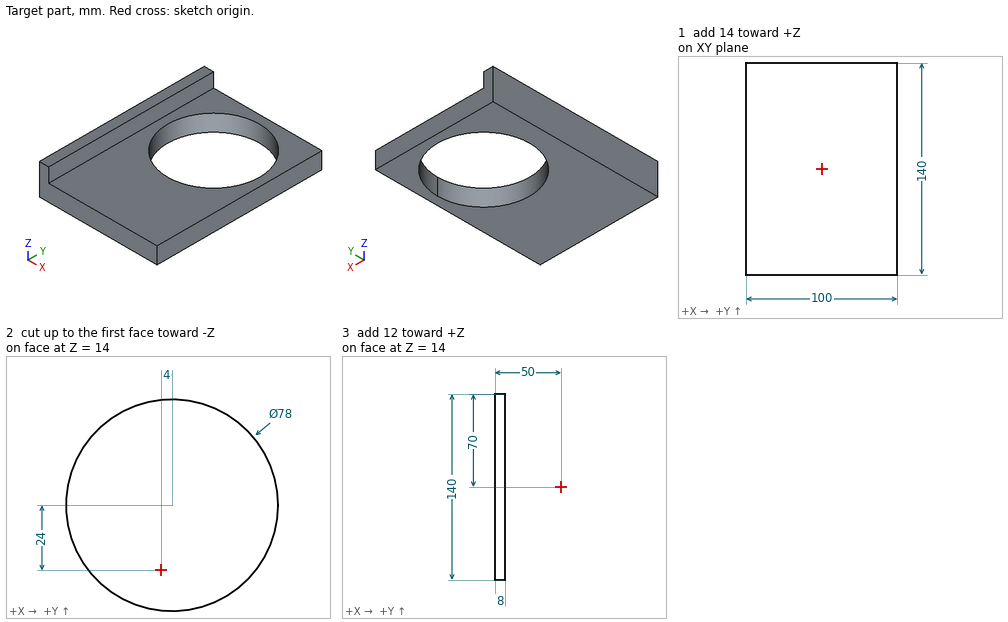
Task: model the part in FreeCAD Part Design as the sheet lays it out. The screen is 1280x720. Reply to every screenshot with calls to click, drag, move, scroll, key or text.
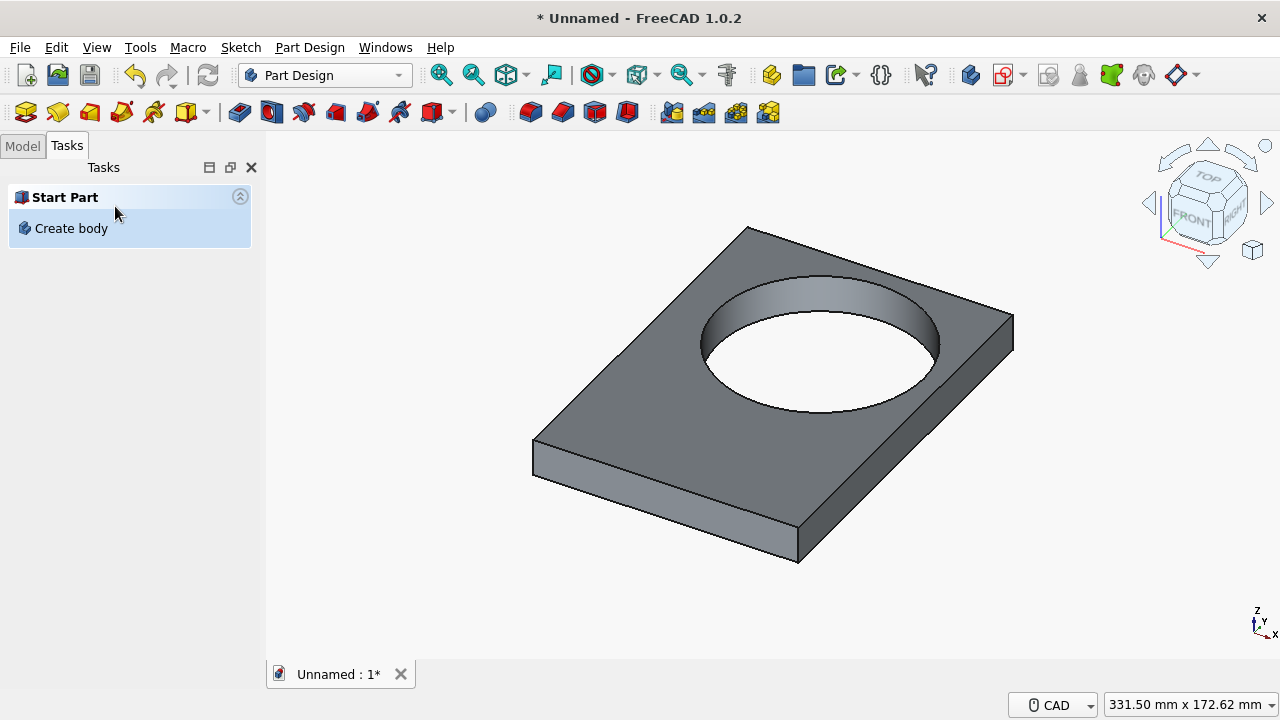
click(674, 425)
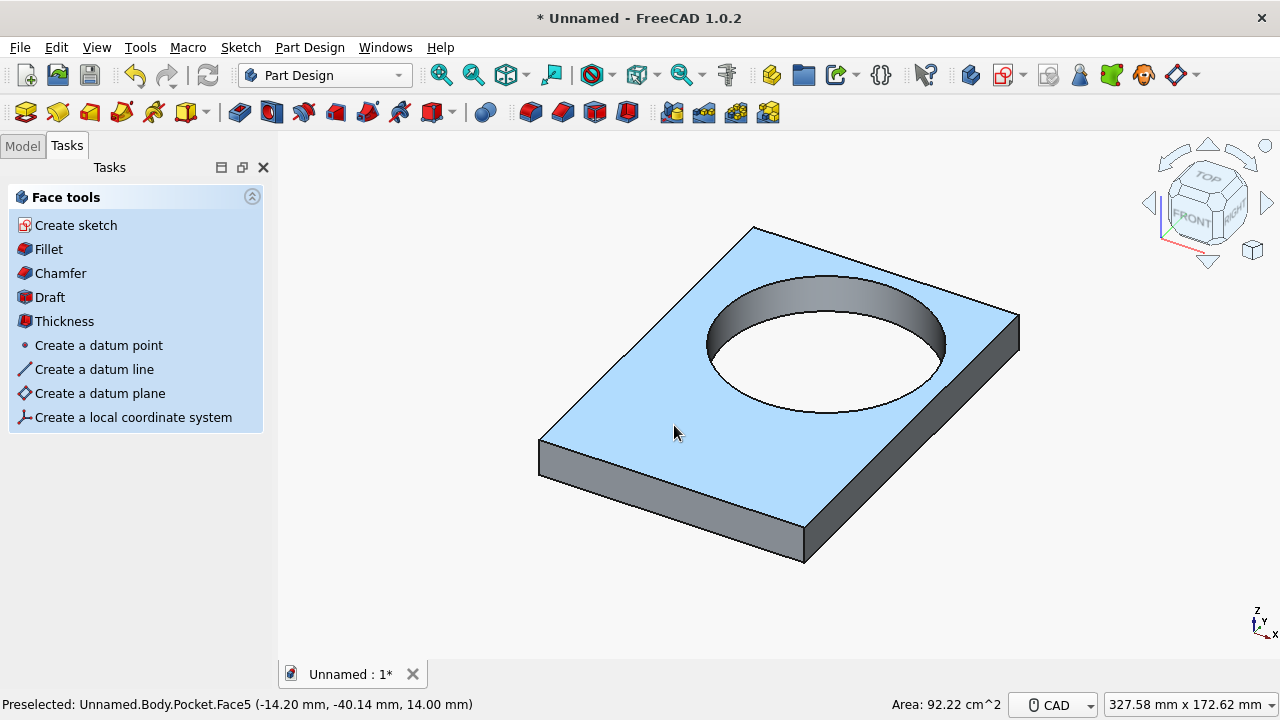
click(1004, 76)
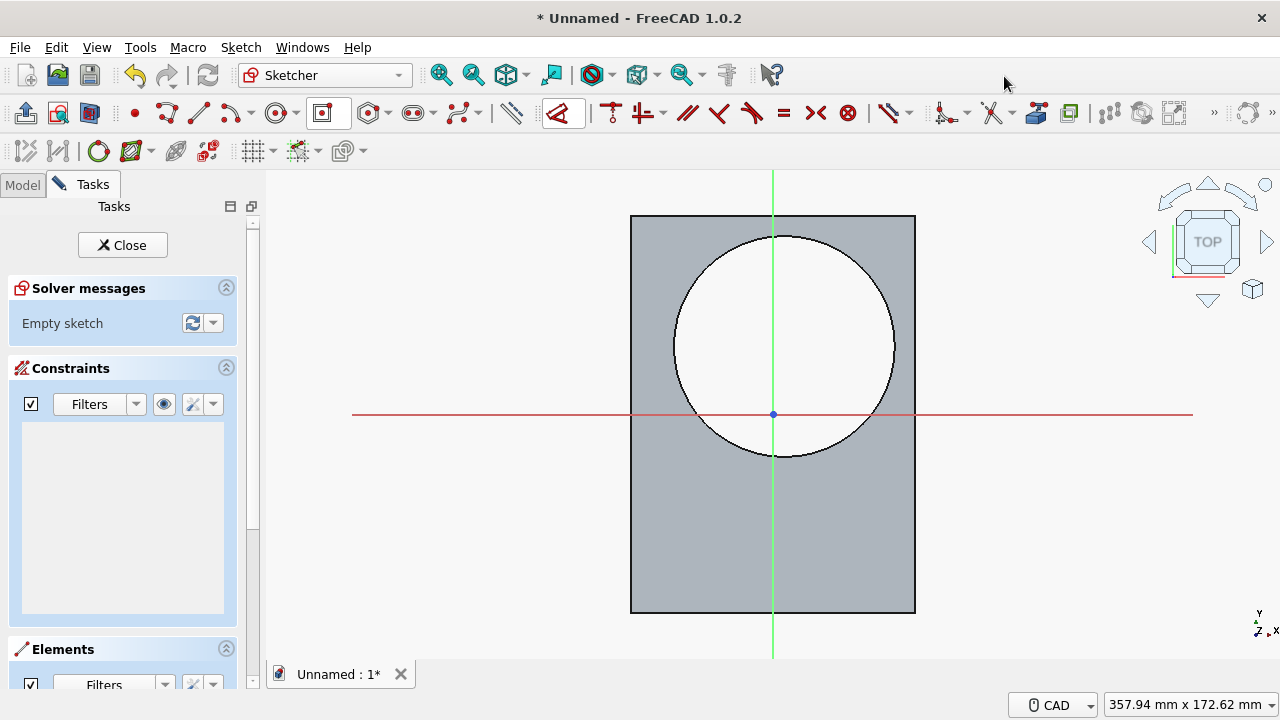
scroll(715, 415, down, 1)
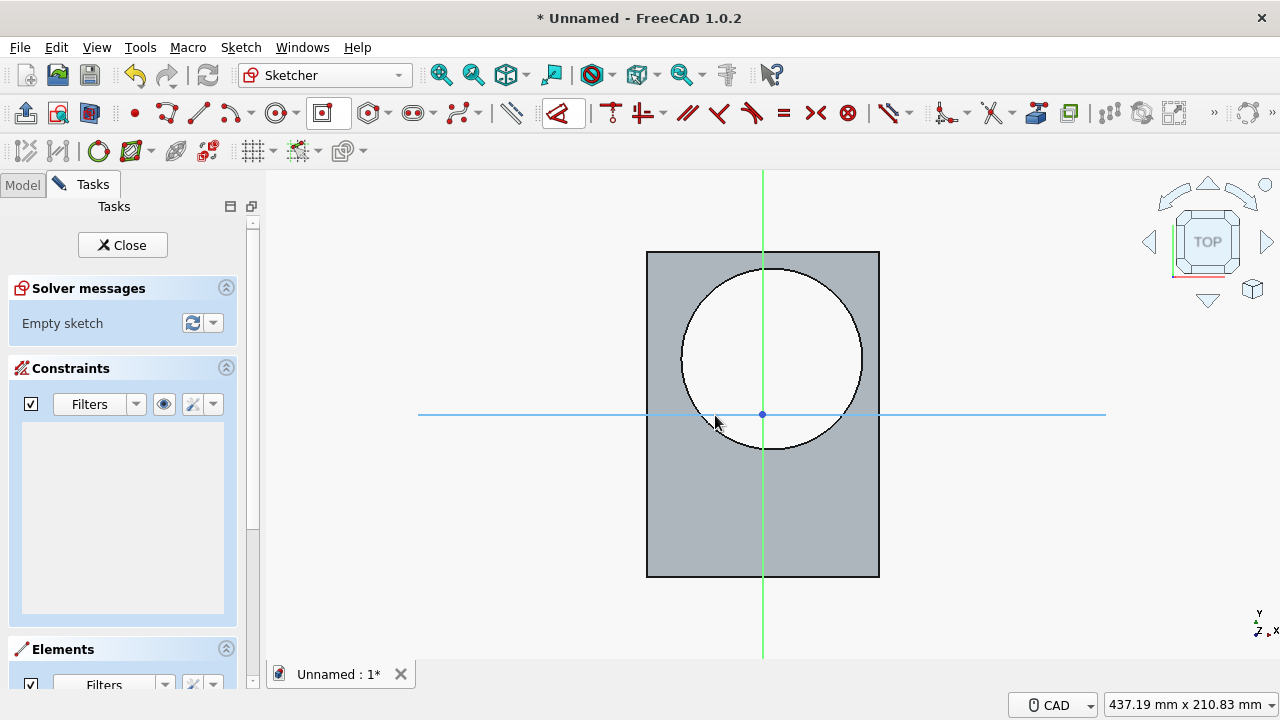
click(346, 114)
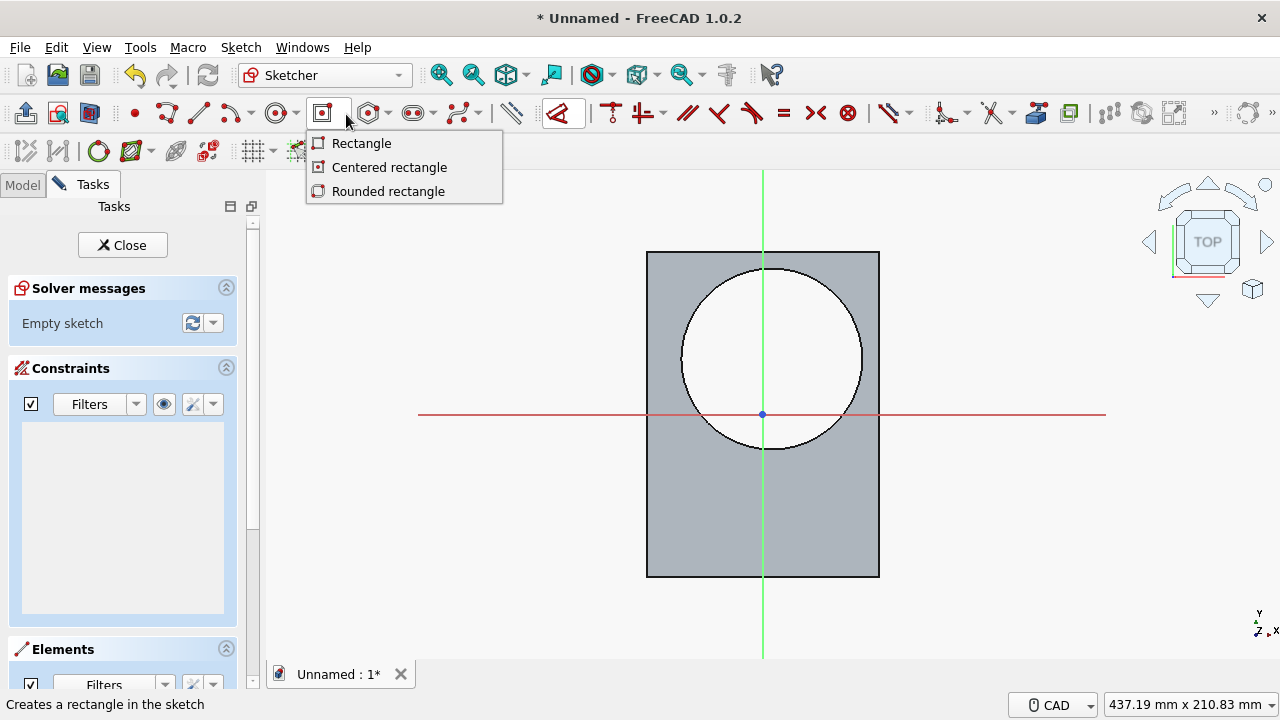
click(404, 143)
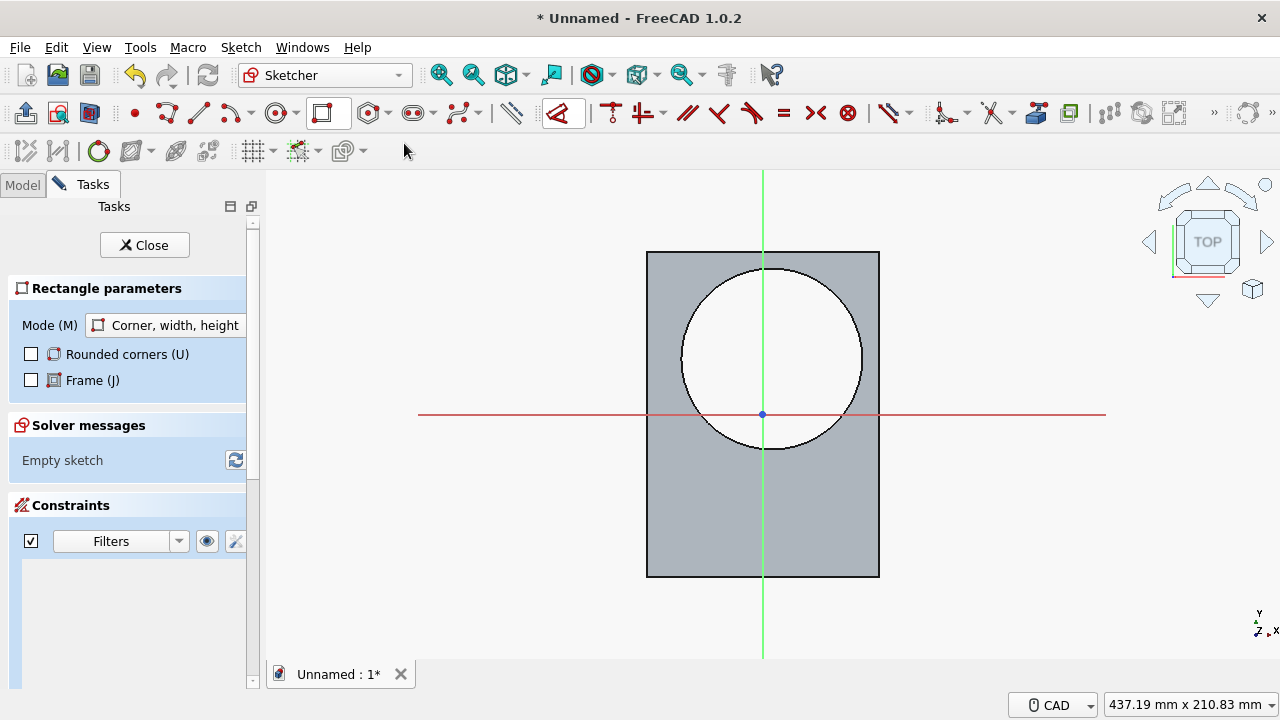
click(647, 252)
move(665, 577)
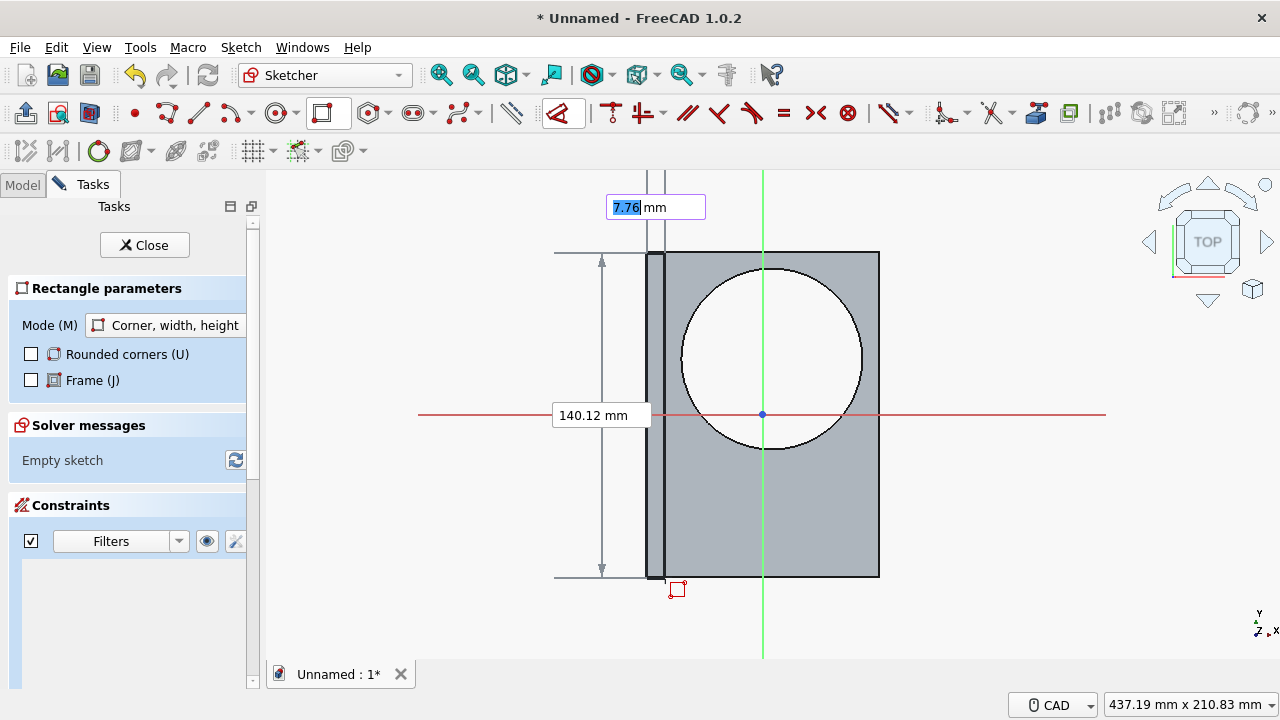
text(8)
key(Tab)
text(140)
key(Return)
key(Escape)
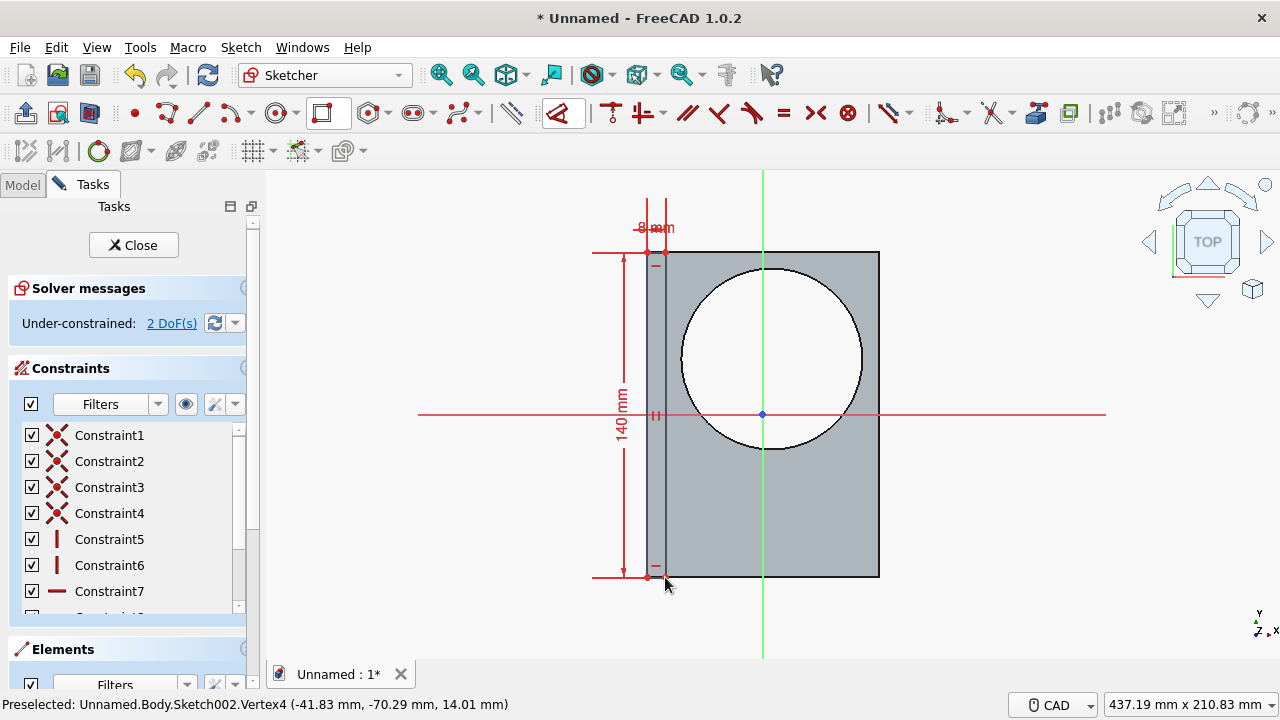
click(647, 253)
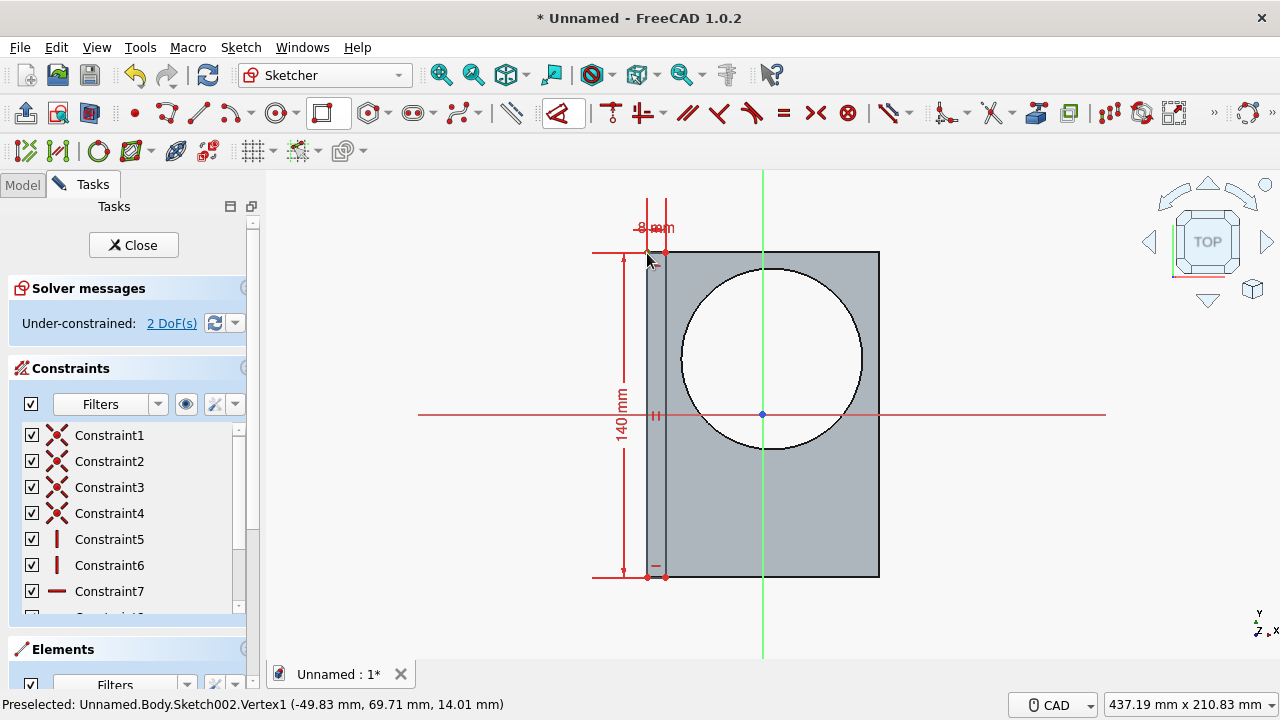
key(l)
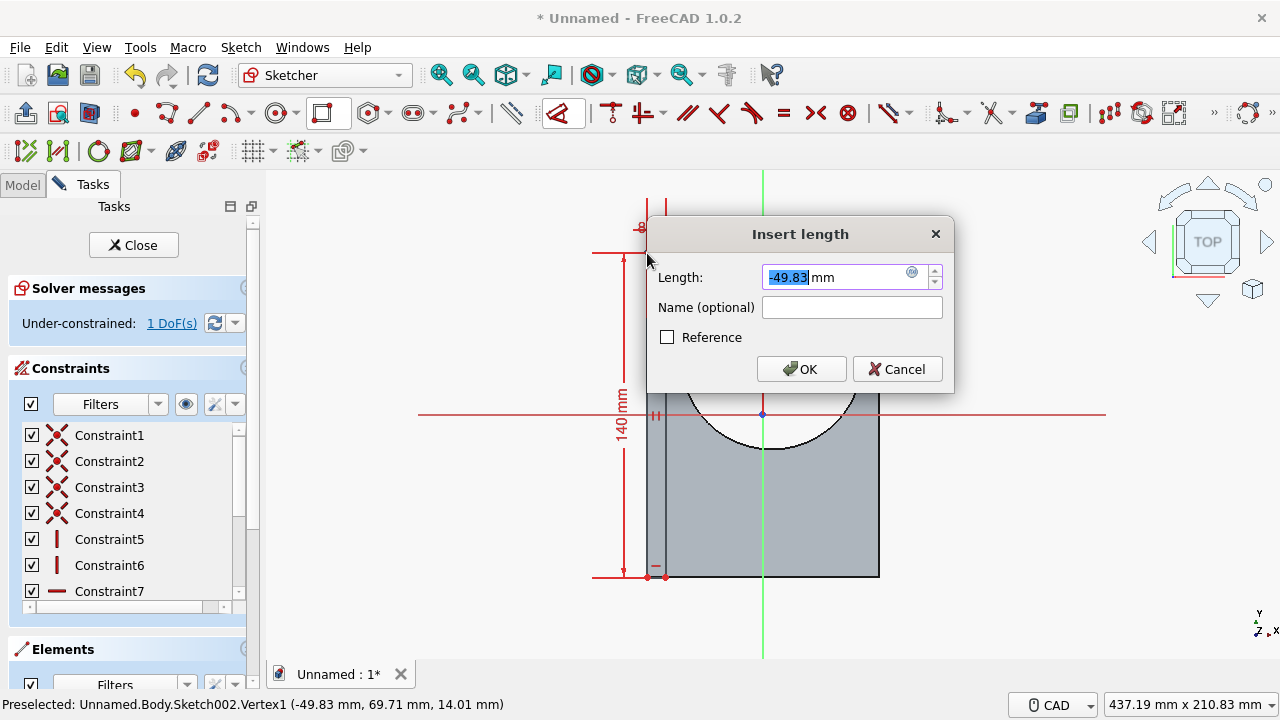
text(-50)
key(Return)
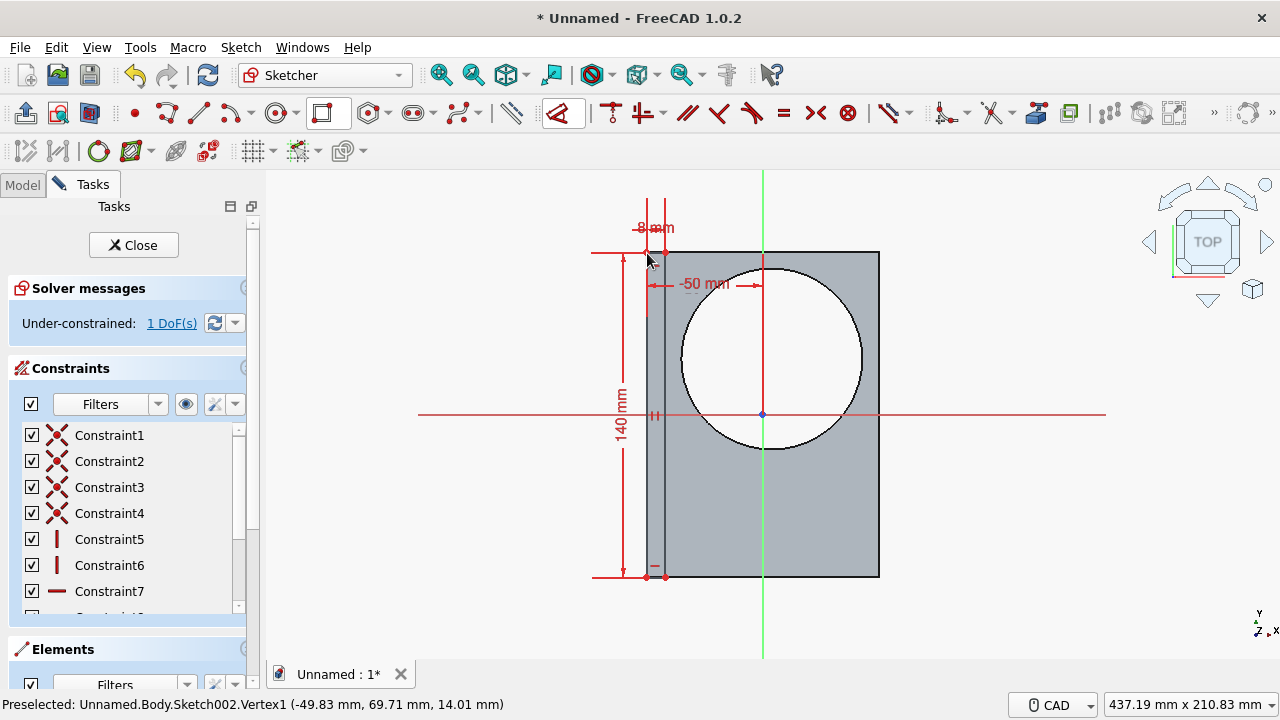
click(647, 253)